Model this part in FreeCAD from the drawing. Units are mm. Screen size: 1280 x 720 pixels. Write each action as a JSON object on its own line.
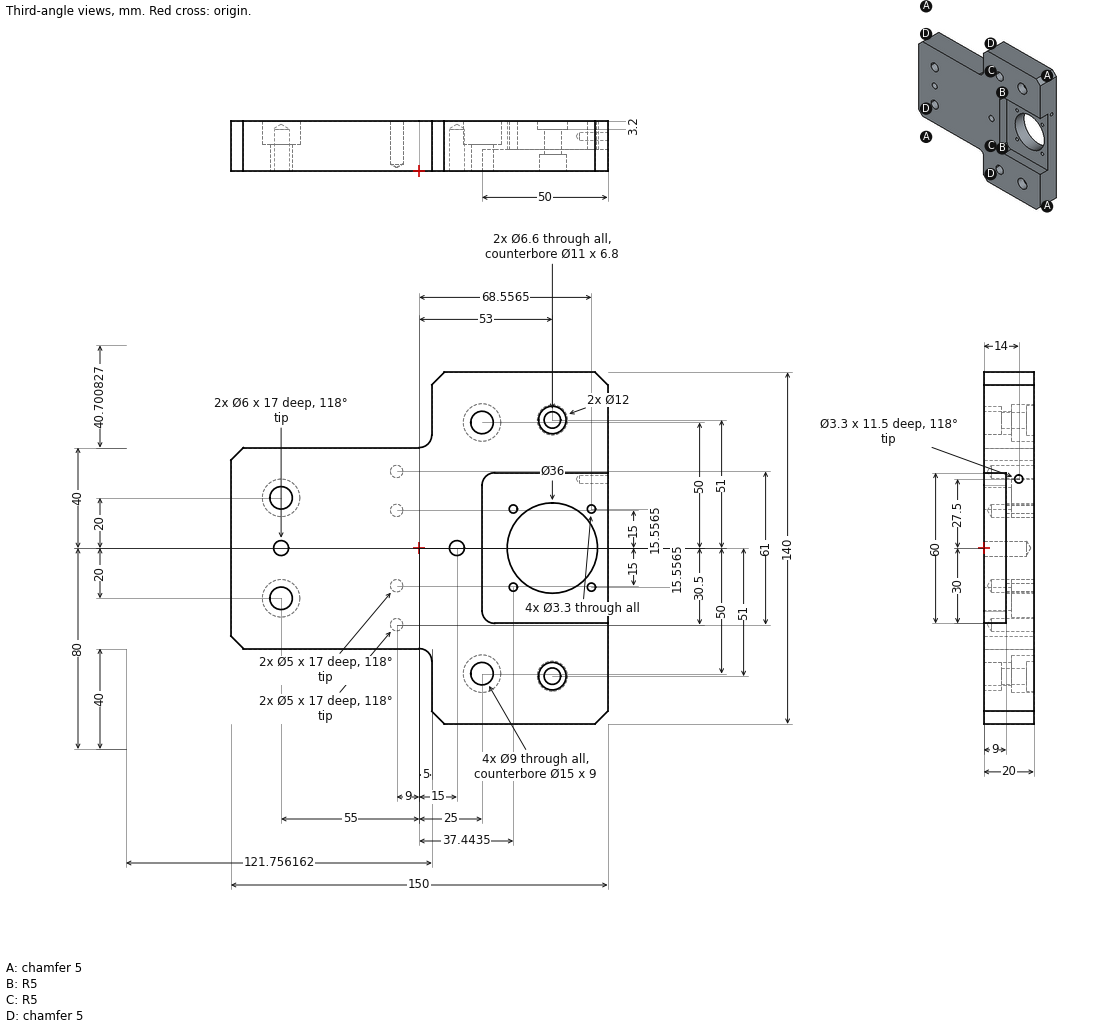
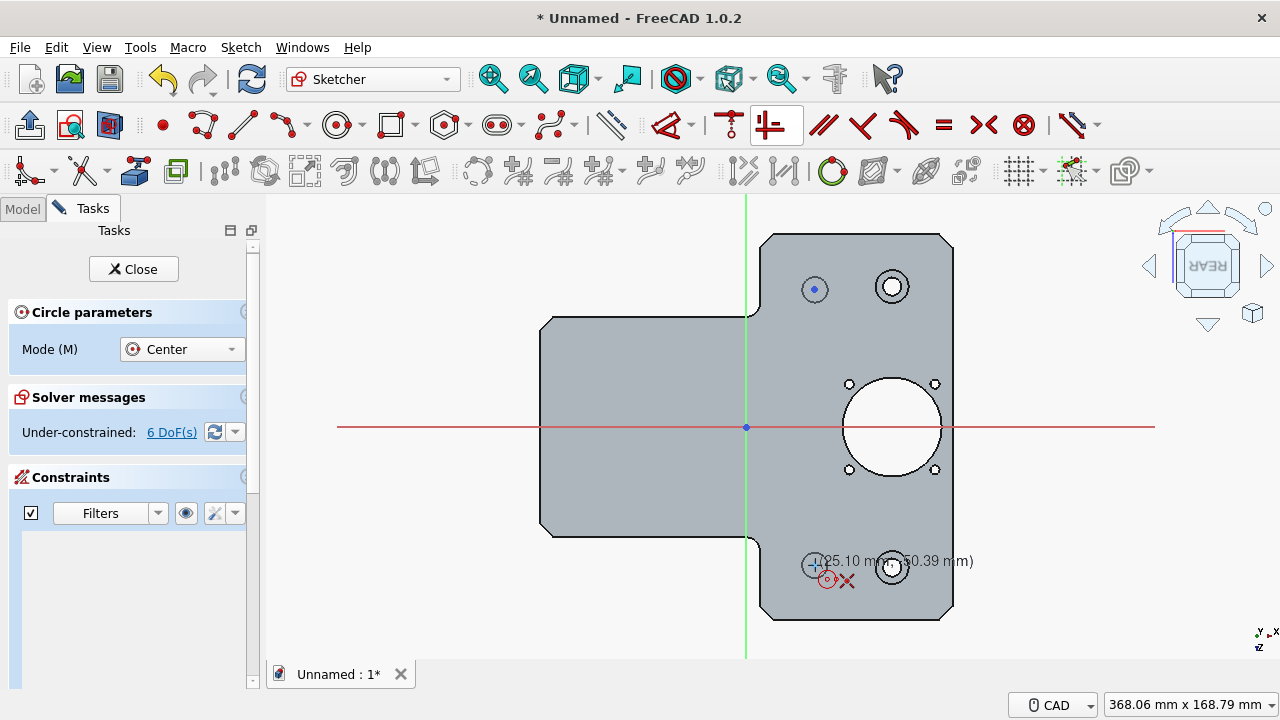
{"action": "scroll", "coordinate": [595, 372], "scroll_direction": "up", "scroll_amount": 4}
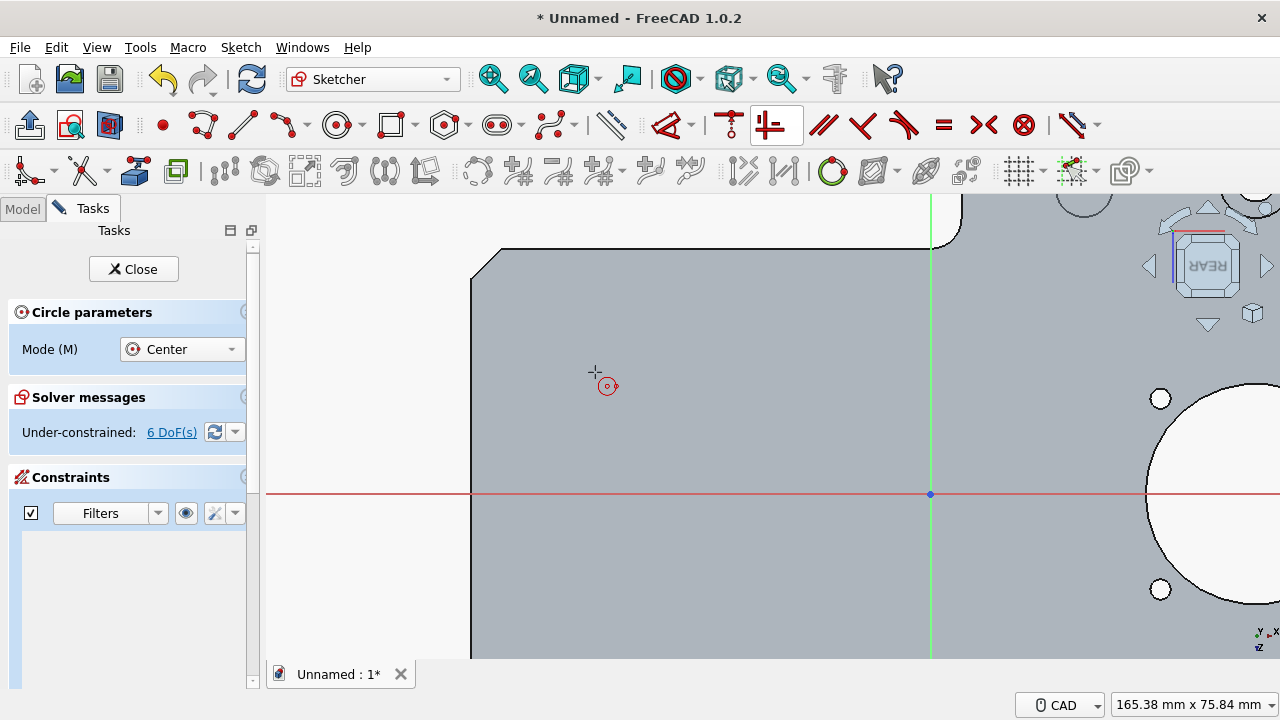
{"action": "left_click", "coordinate": [594, 371]}
{"action": "left_click", "coordinate": [613, 352]}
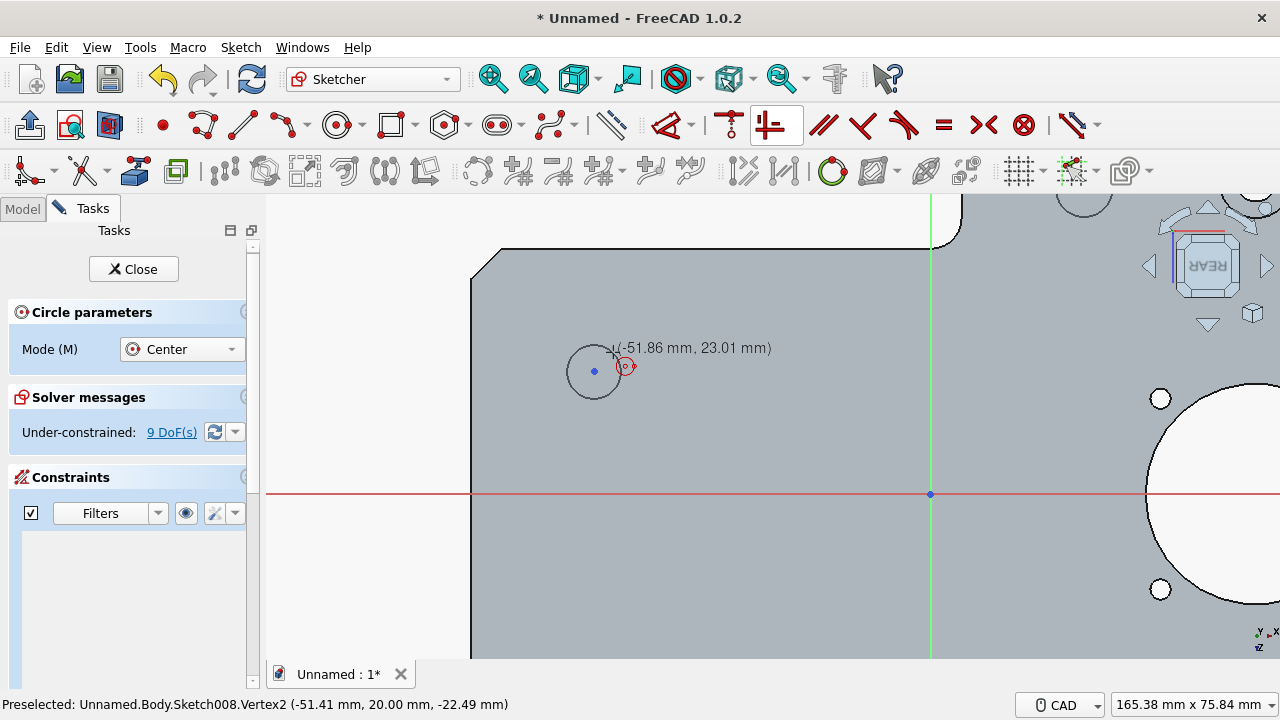
{"action": "left_click", "coordinate": [594, 617]}
{"action": "left_click", "coordinate": [613, 597]}
{"action": "key", "text": "Escape"}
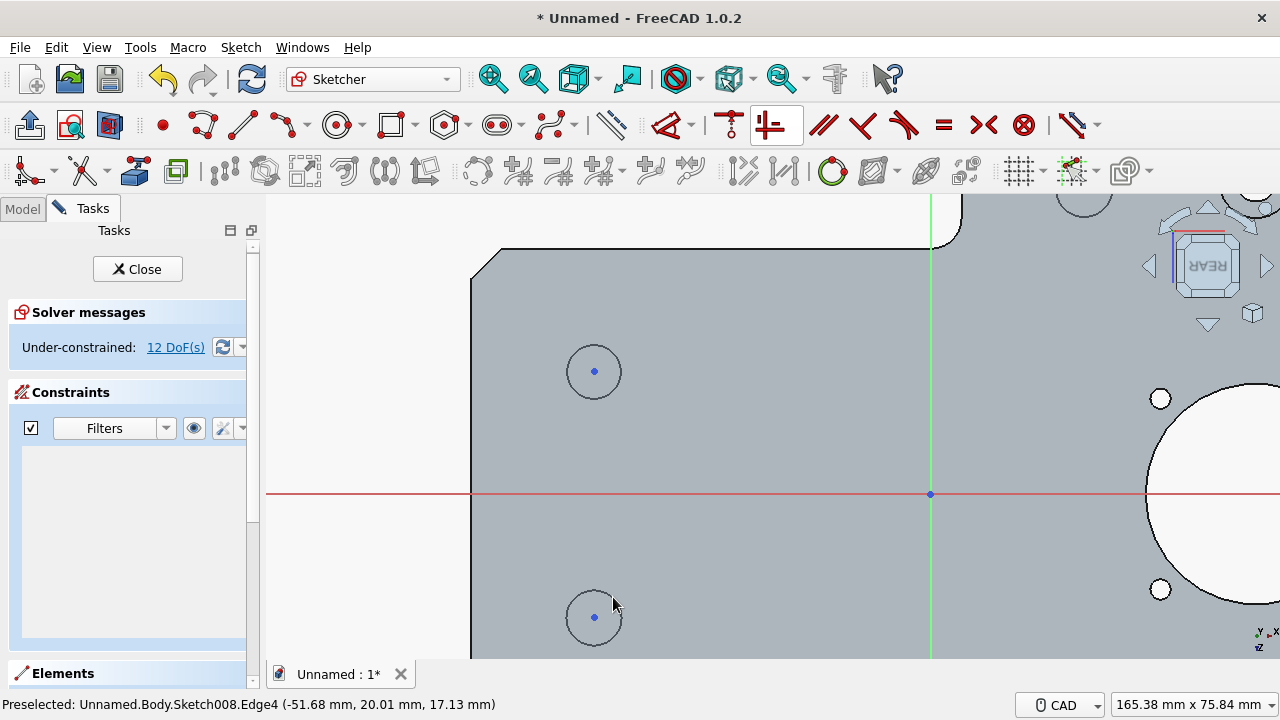
{"action": "scroll", "coordinate": [595, 371], "scroll_direction": "down", "scroll_amount": 4}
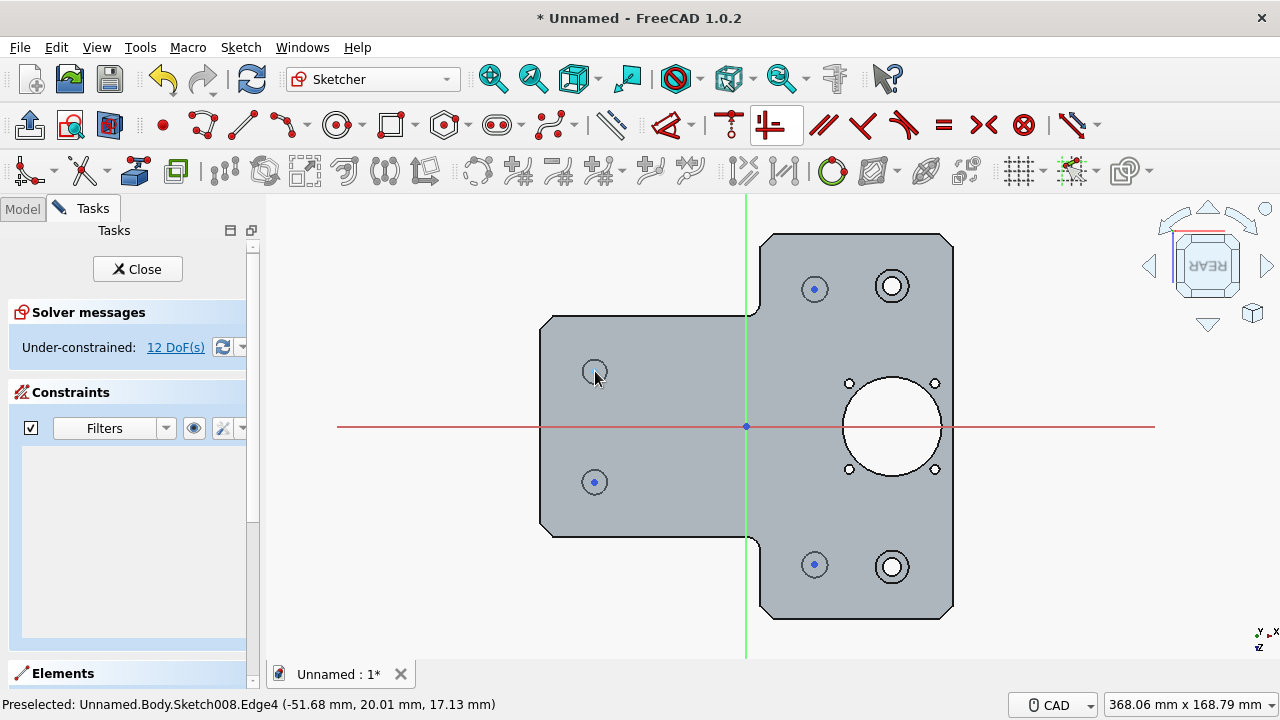
{"action": "left_click", "coordinate": [824, 280]}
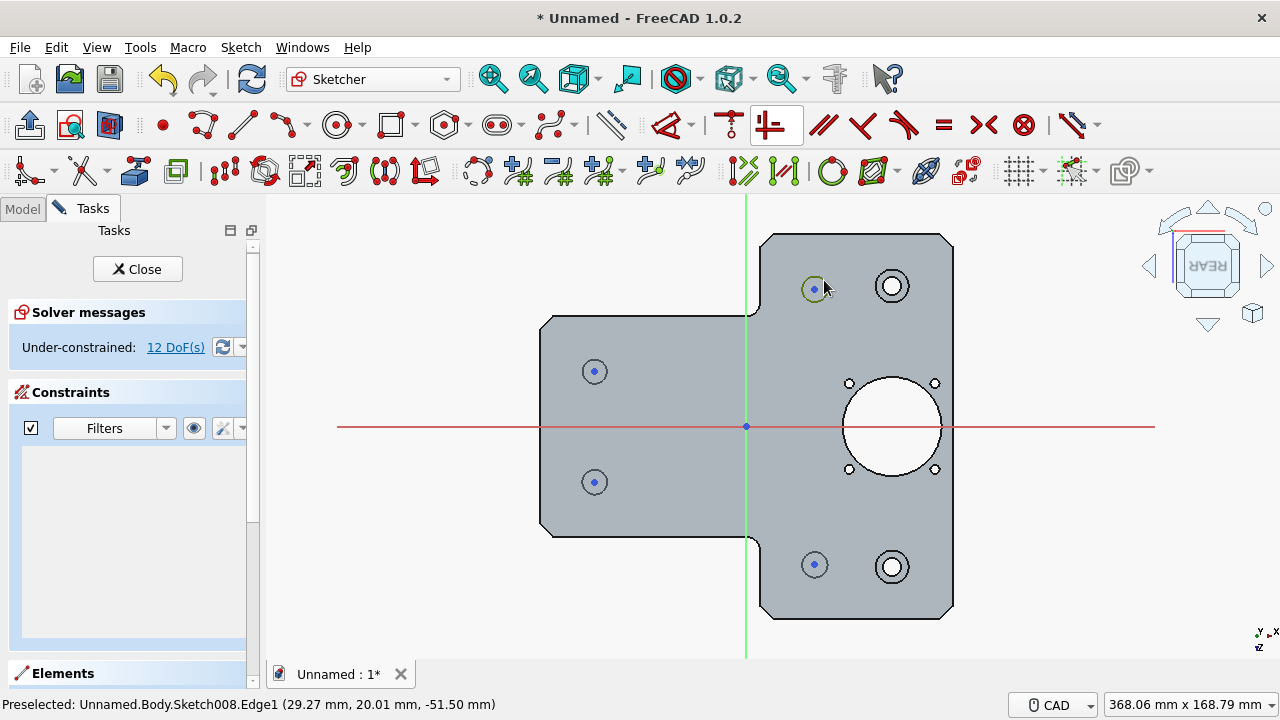
{"action": "left_click", "coordinate": [824, 556]}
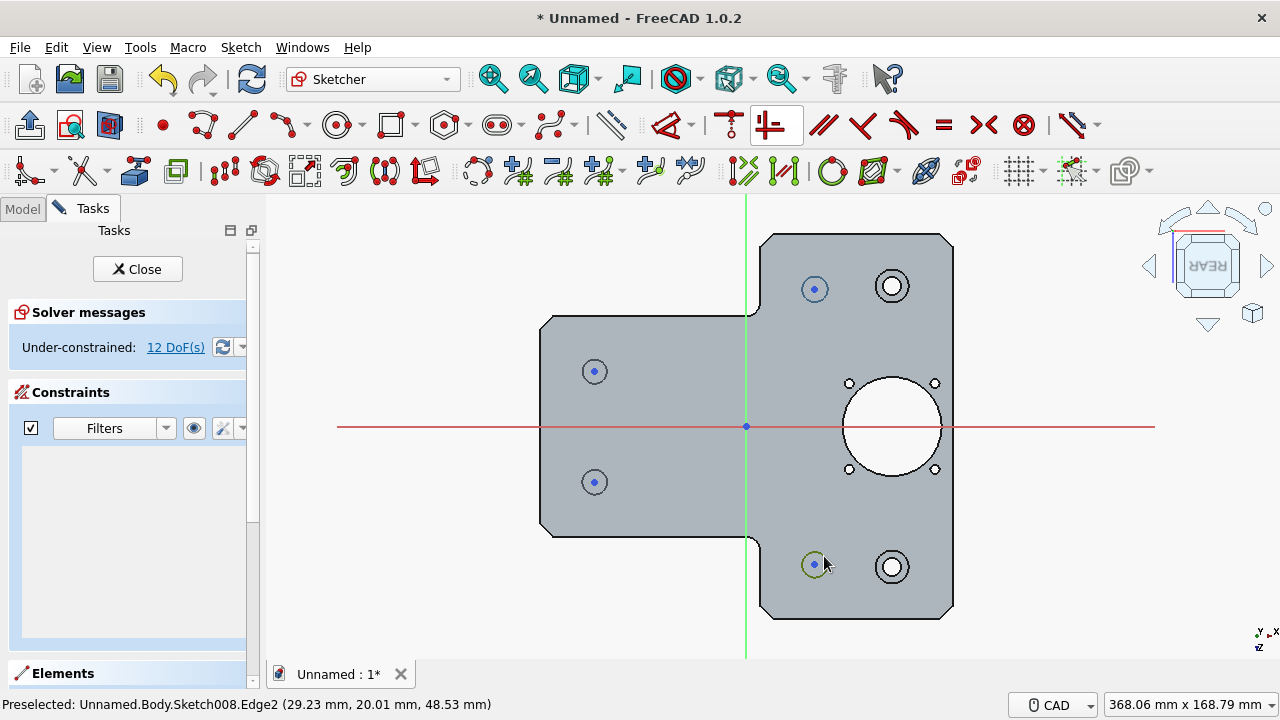
{"action": "left_click", "coordinate": [603, 363]}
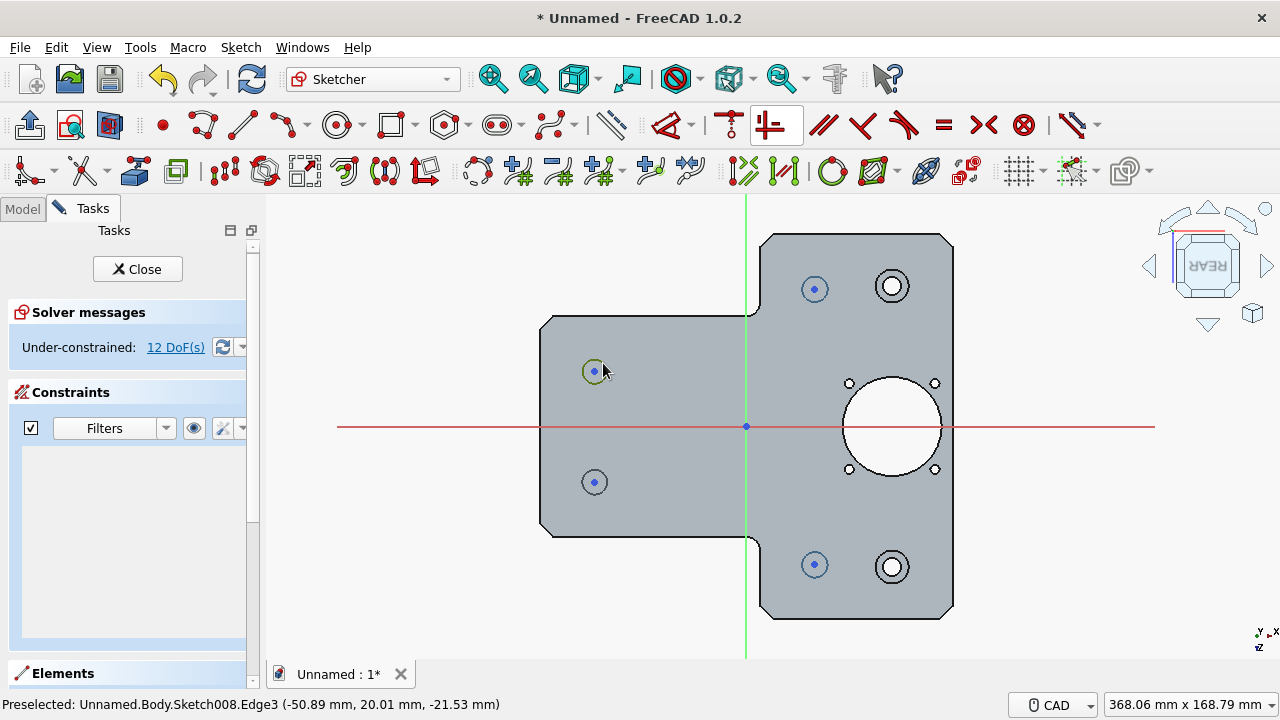
{"action": "left_click", "coordinate": [603, 473]}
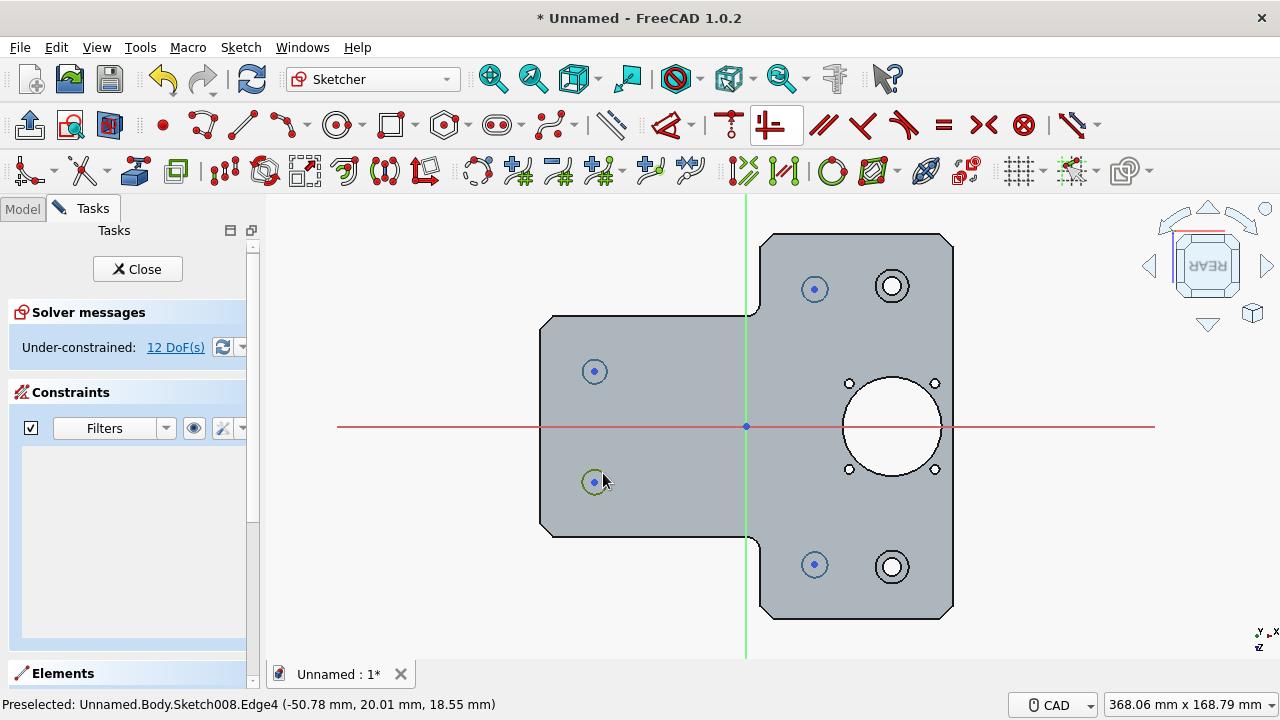
{"action": "left_click", "coordinate": [944, 126]}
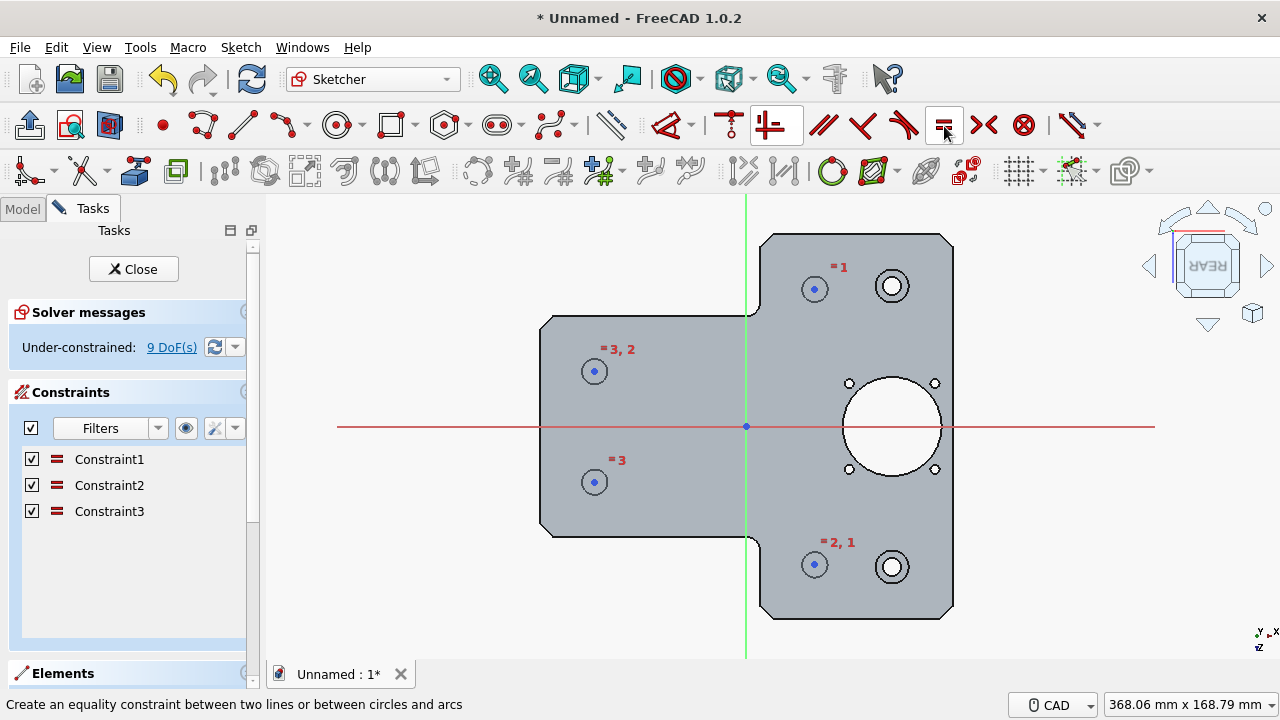
{"action": "left_click", "coordinate": [815, 289]}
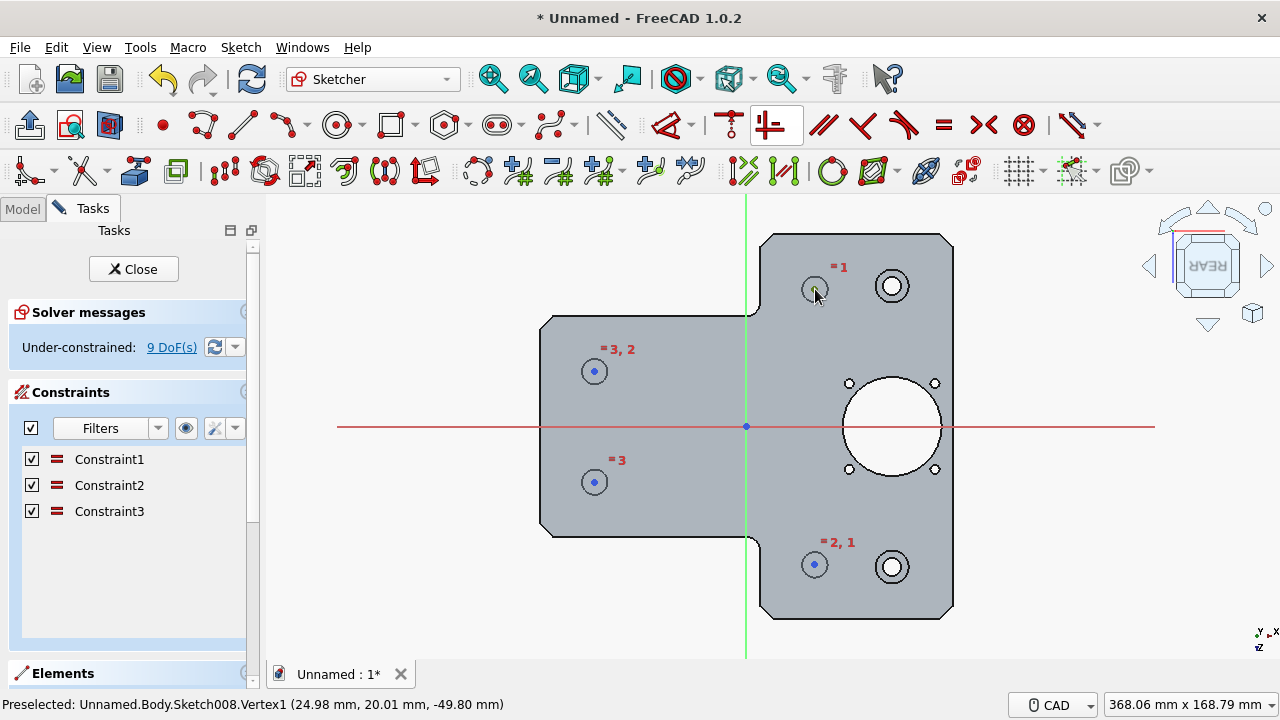
{"action": "left_click", "coordinate": [815, 565]}